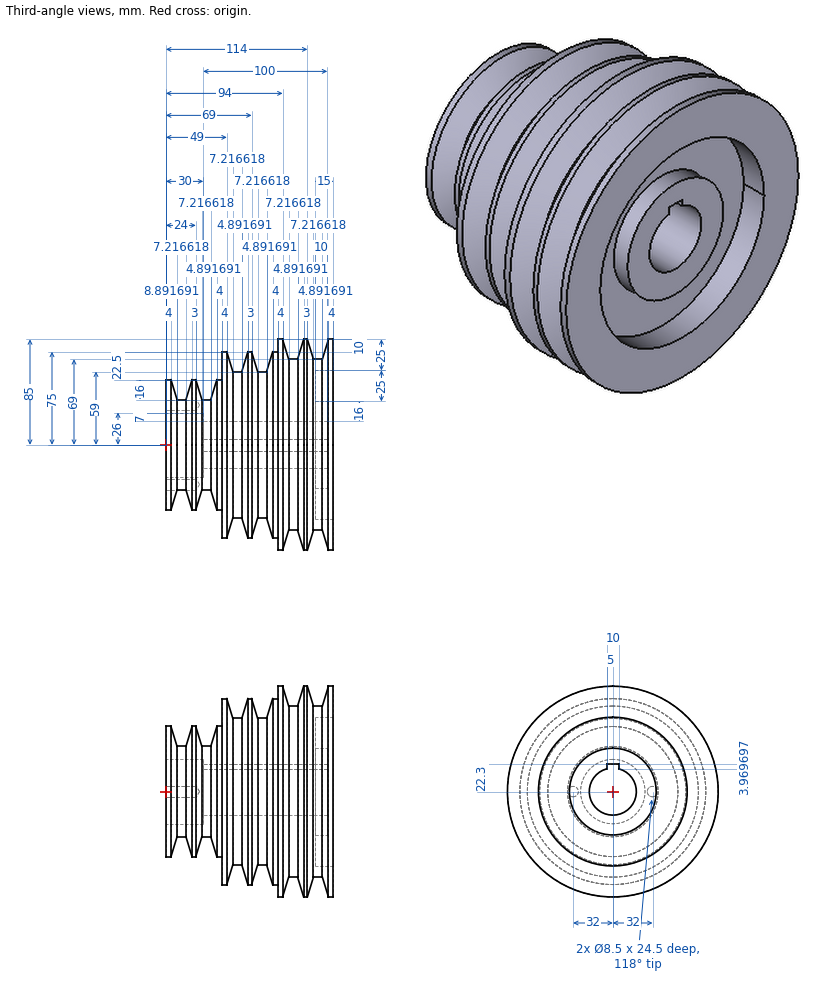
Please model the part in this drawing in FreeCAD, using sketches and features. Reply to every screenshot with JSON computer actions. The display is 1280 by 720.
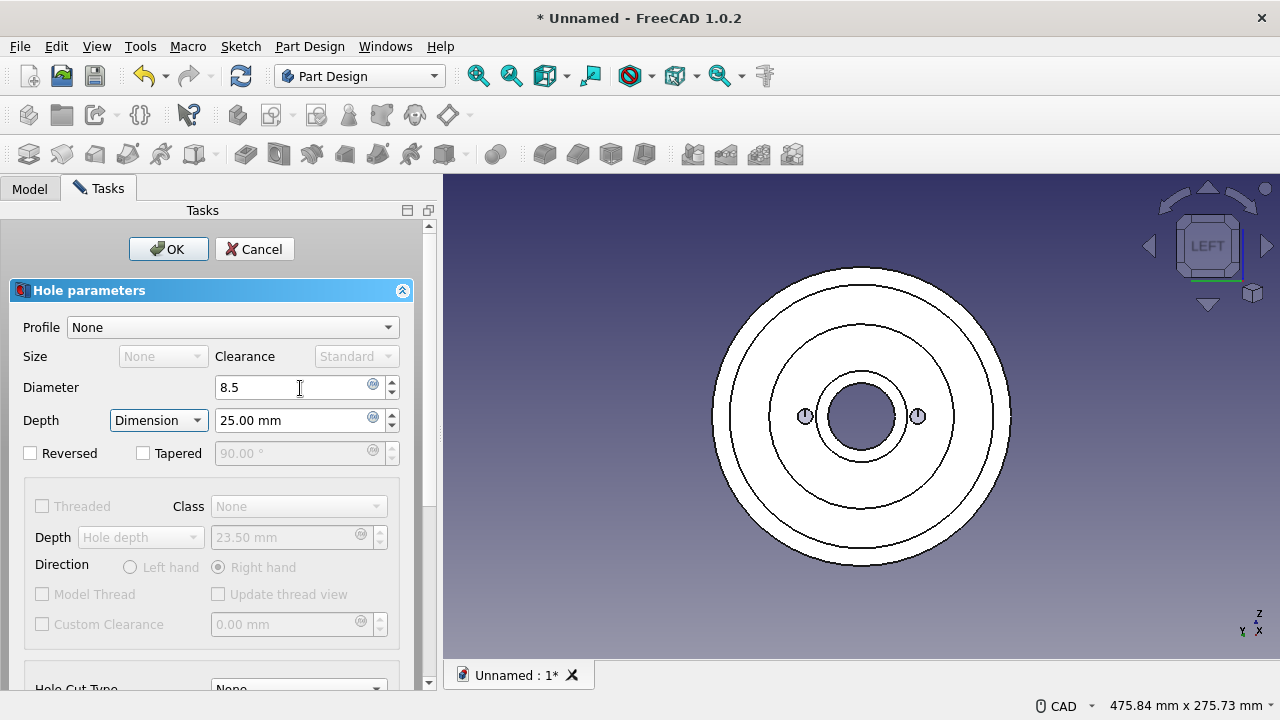
{"action": "triple_click", "coordinate": [300, 420]}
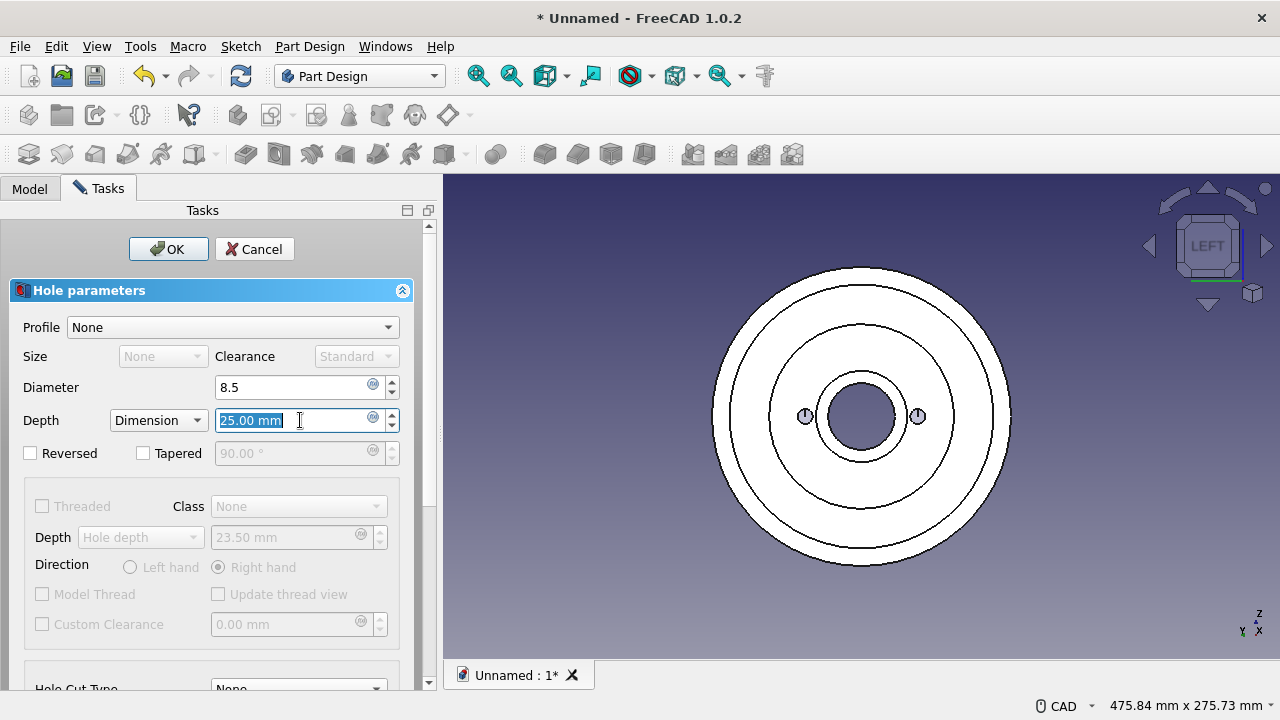
{"action": "type", "text": "24.5"}
{"action": "key", "text": "Tab"}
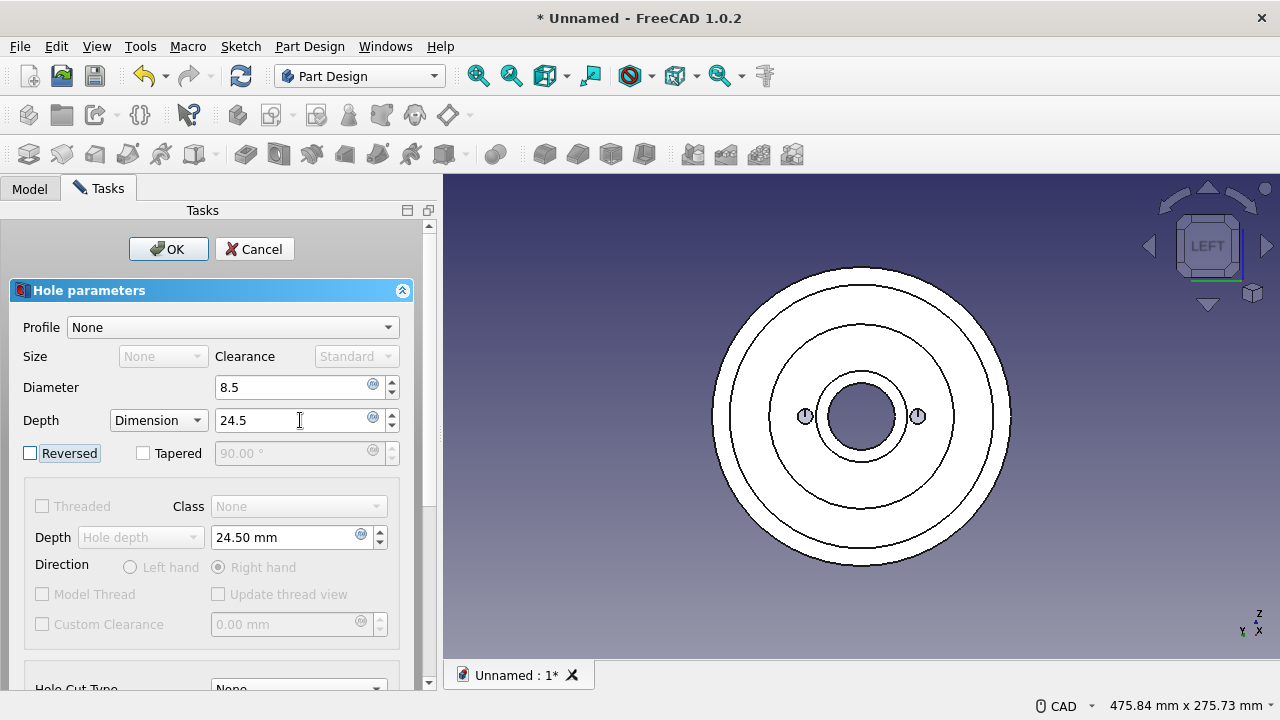
{"action": "left_click", "coordinate": [169, 249]}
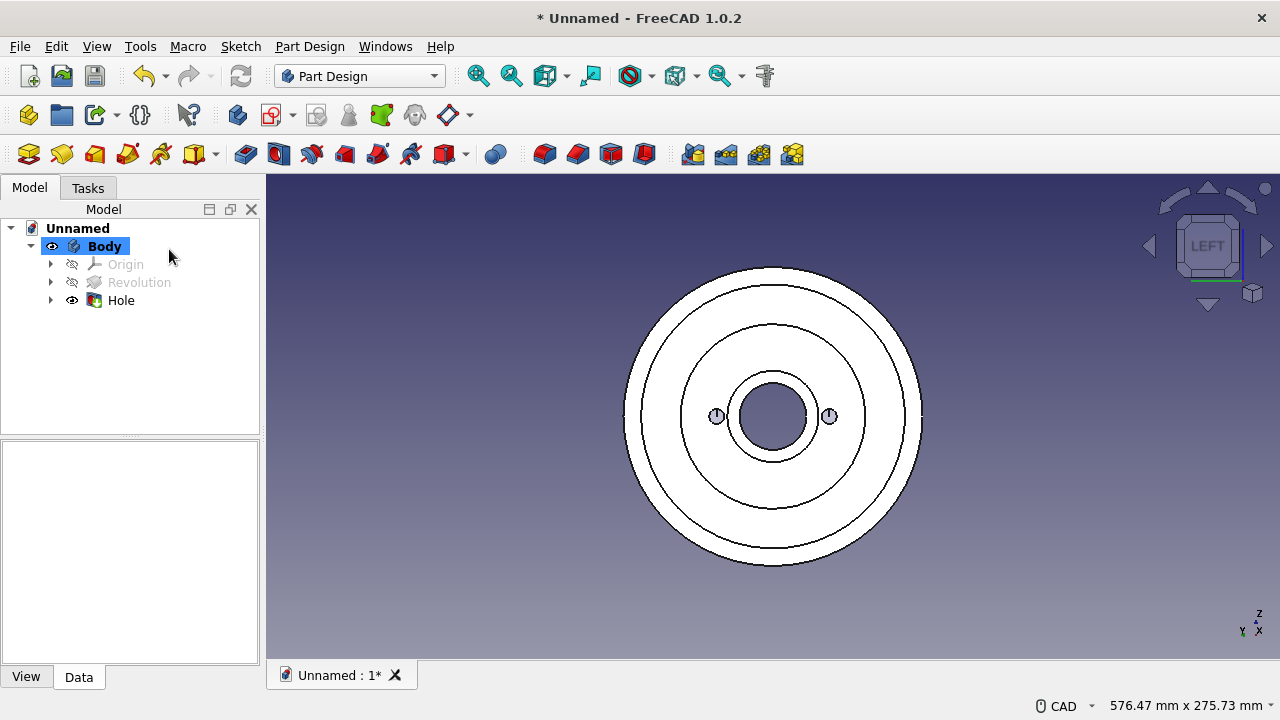
{"action": "key", "text": "0"}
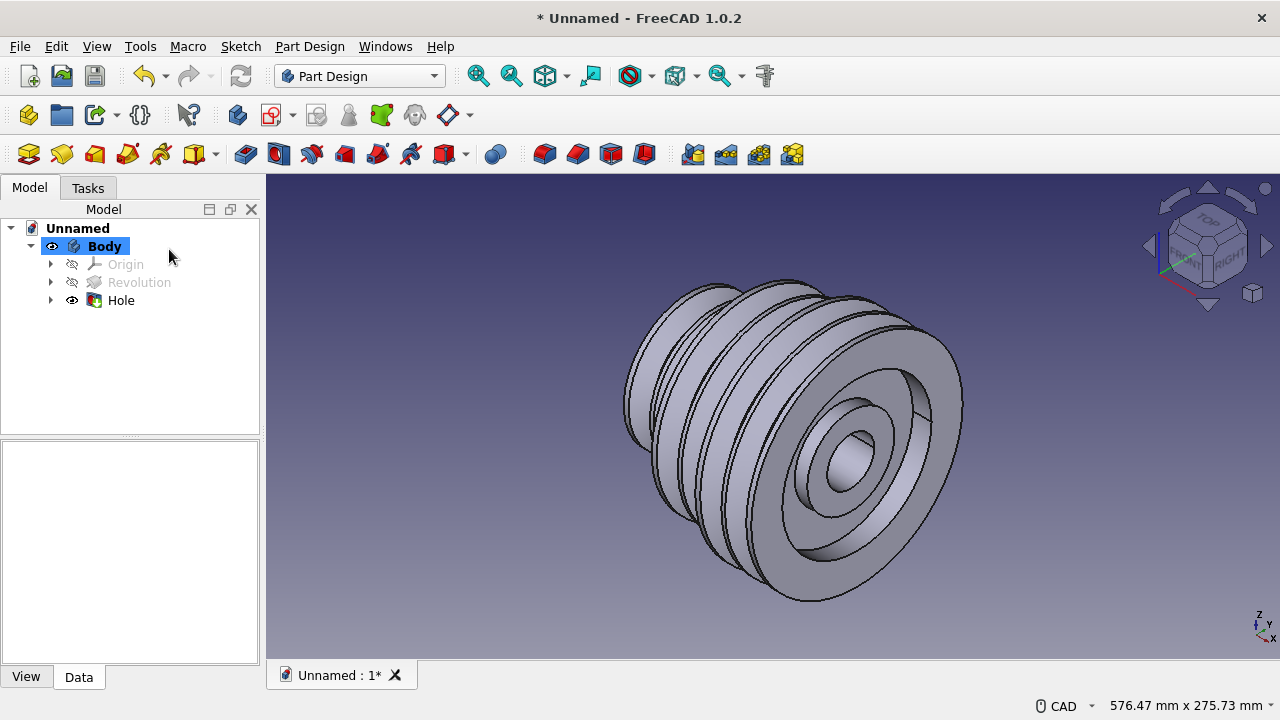
{"action": "left_click", "coordinate": [826, 503]}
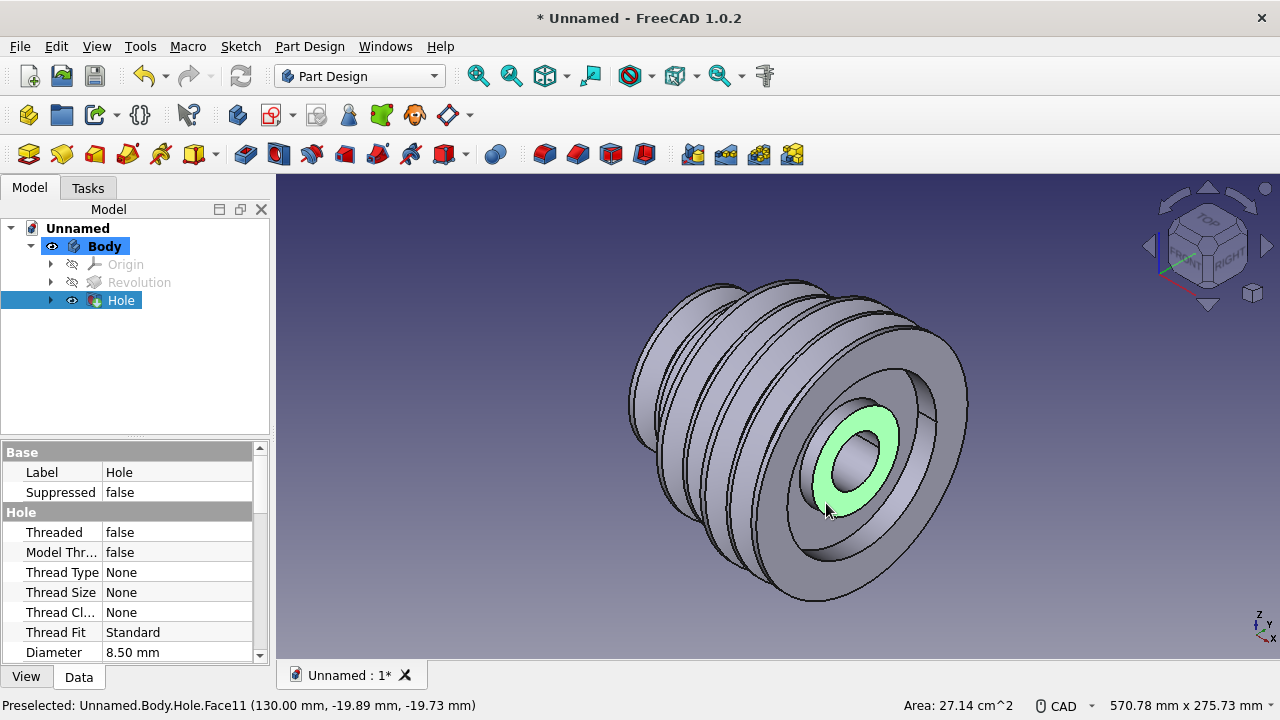
{"action": "left_click", "coordinate": [270, 116]}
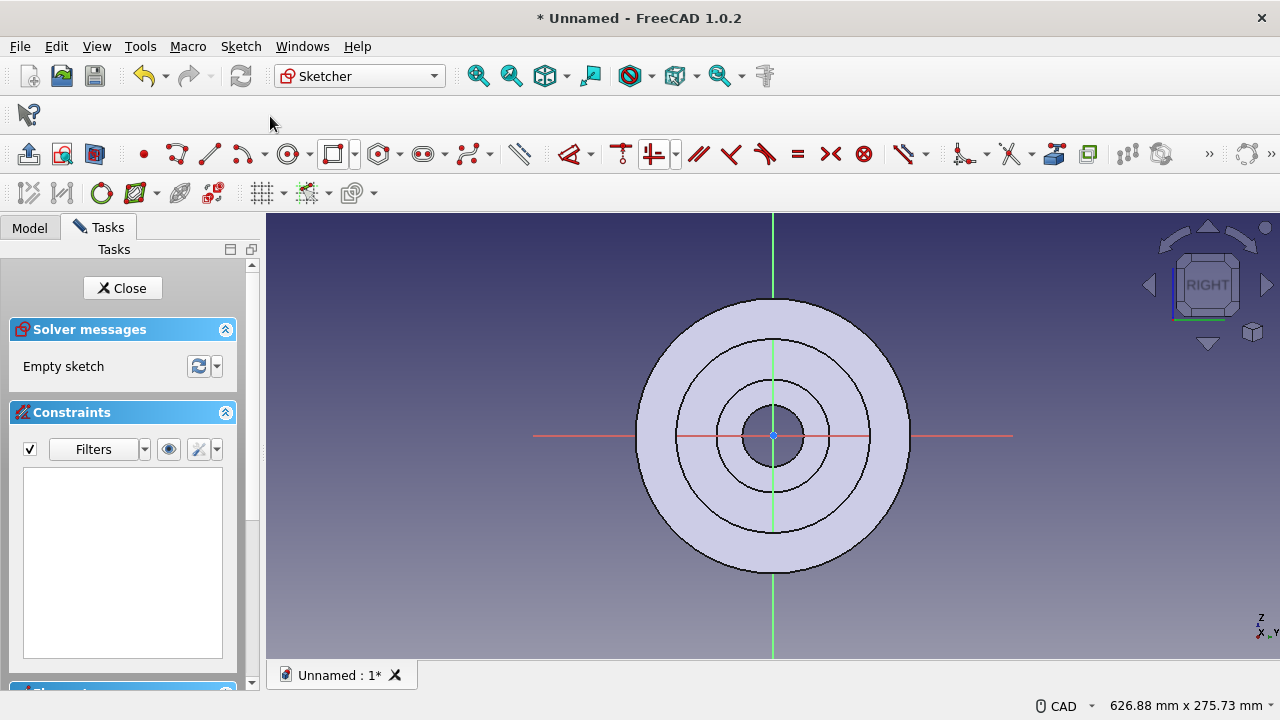
{"action": "left_click", "coordinate": [95, 154]}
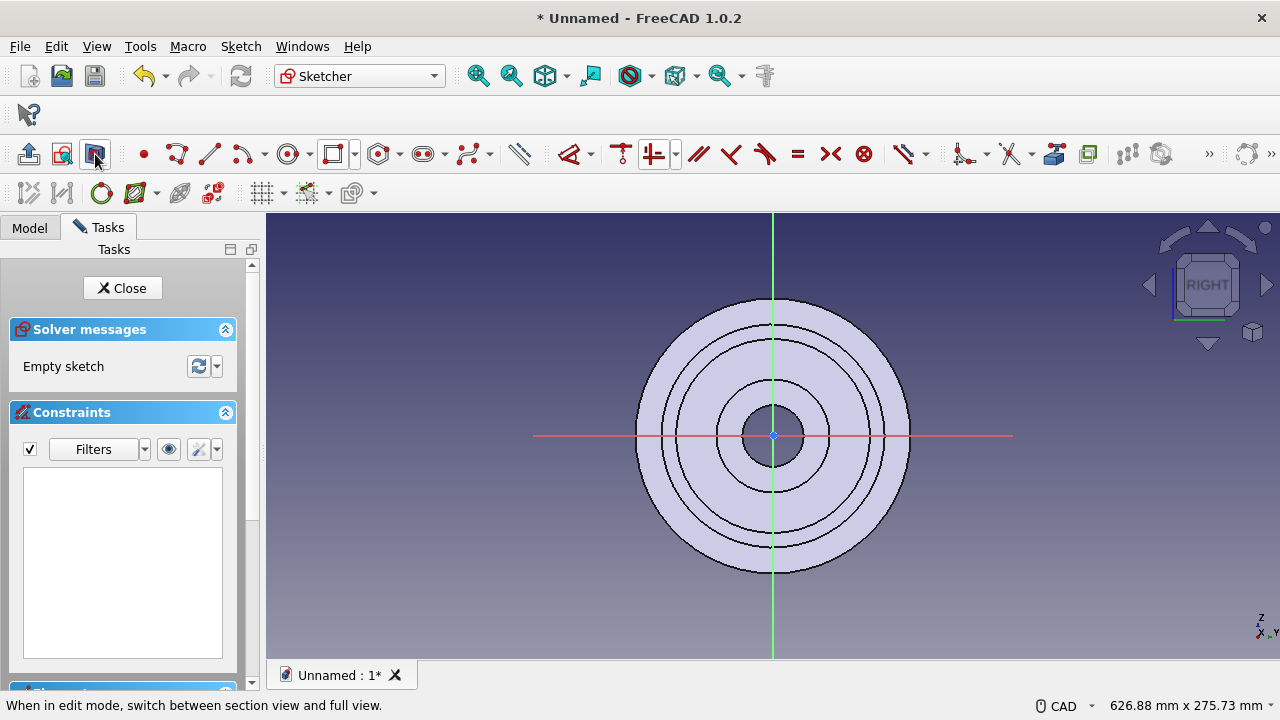
{"action": "scroll", "coordinate": [784, 415], "scroll_direction": "up", "scroll_amount": 10}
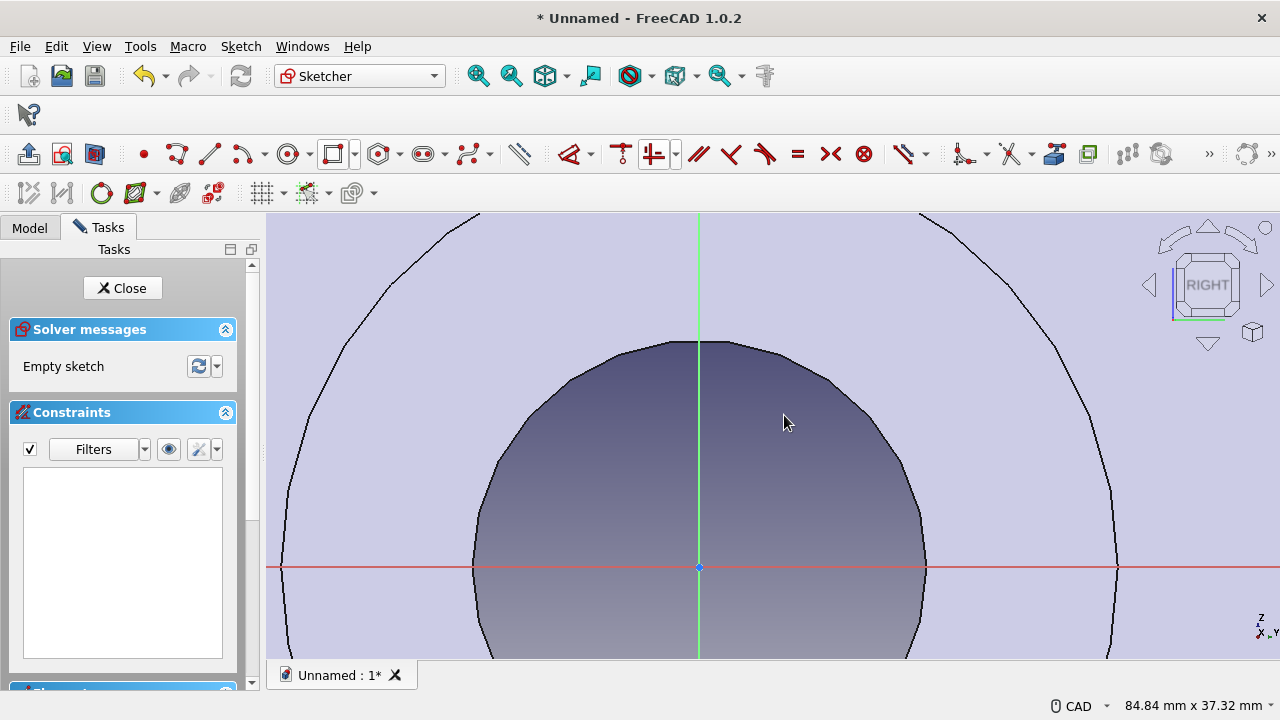
{"action": "left_click", "coordinate": [332, 154]}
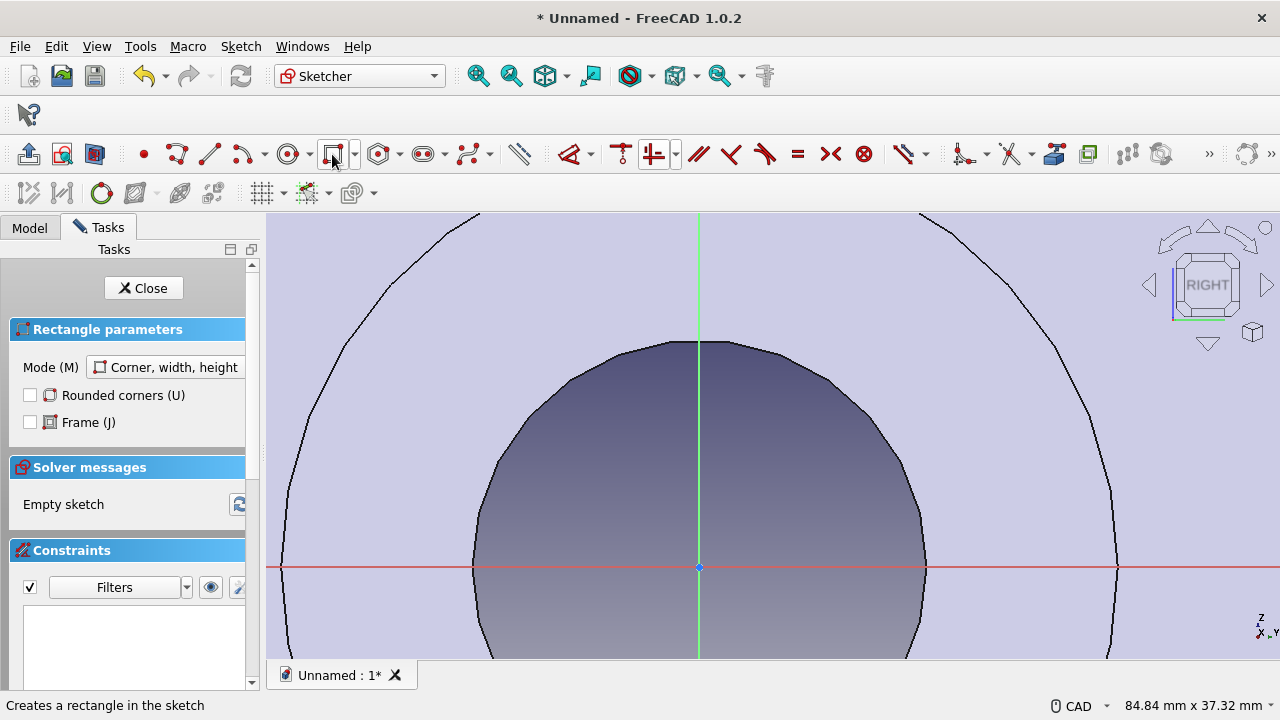
{"action": "left_click", "coordinate": [640, 301]}
{"action": "mouse_move", "coordinate": [759, 348]}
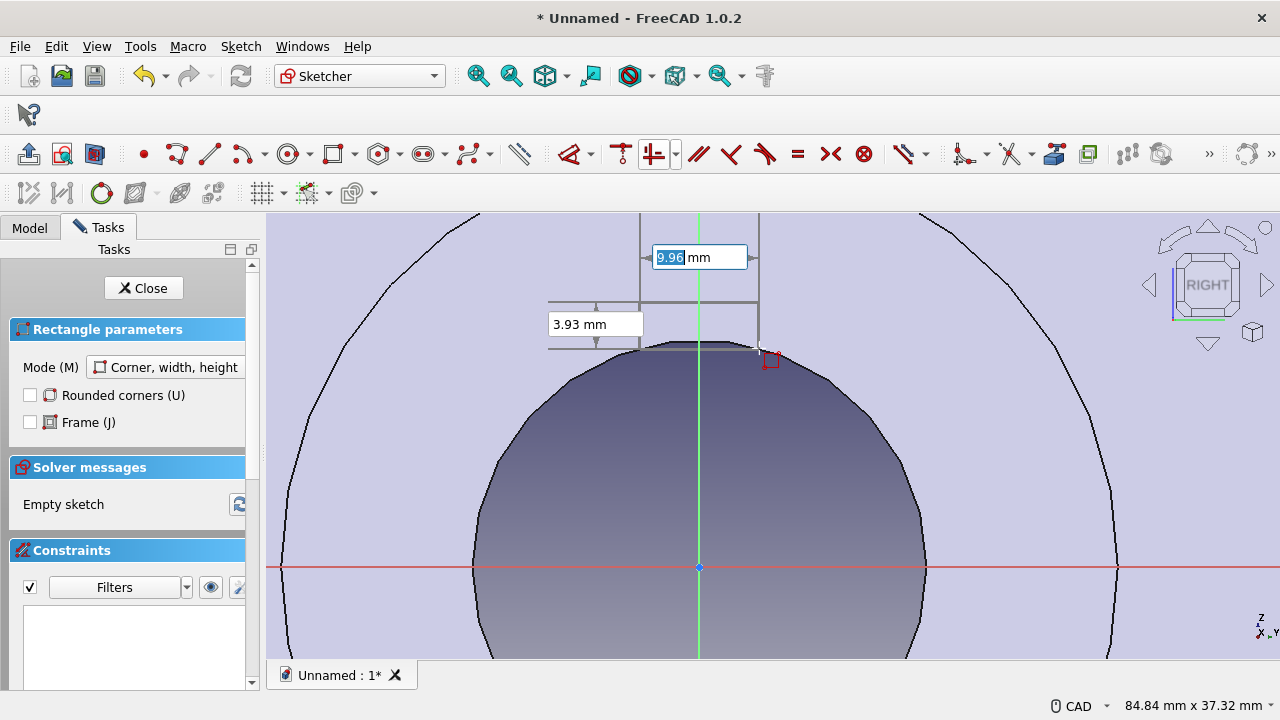
{"action": "type", "text": "10"}
{"action": "key", "text": "Tab"}
{"action": "type", "text": "3.969697"}
{"action": "key", "text": "Return"}
{"action": "key", "text": "Escape"}